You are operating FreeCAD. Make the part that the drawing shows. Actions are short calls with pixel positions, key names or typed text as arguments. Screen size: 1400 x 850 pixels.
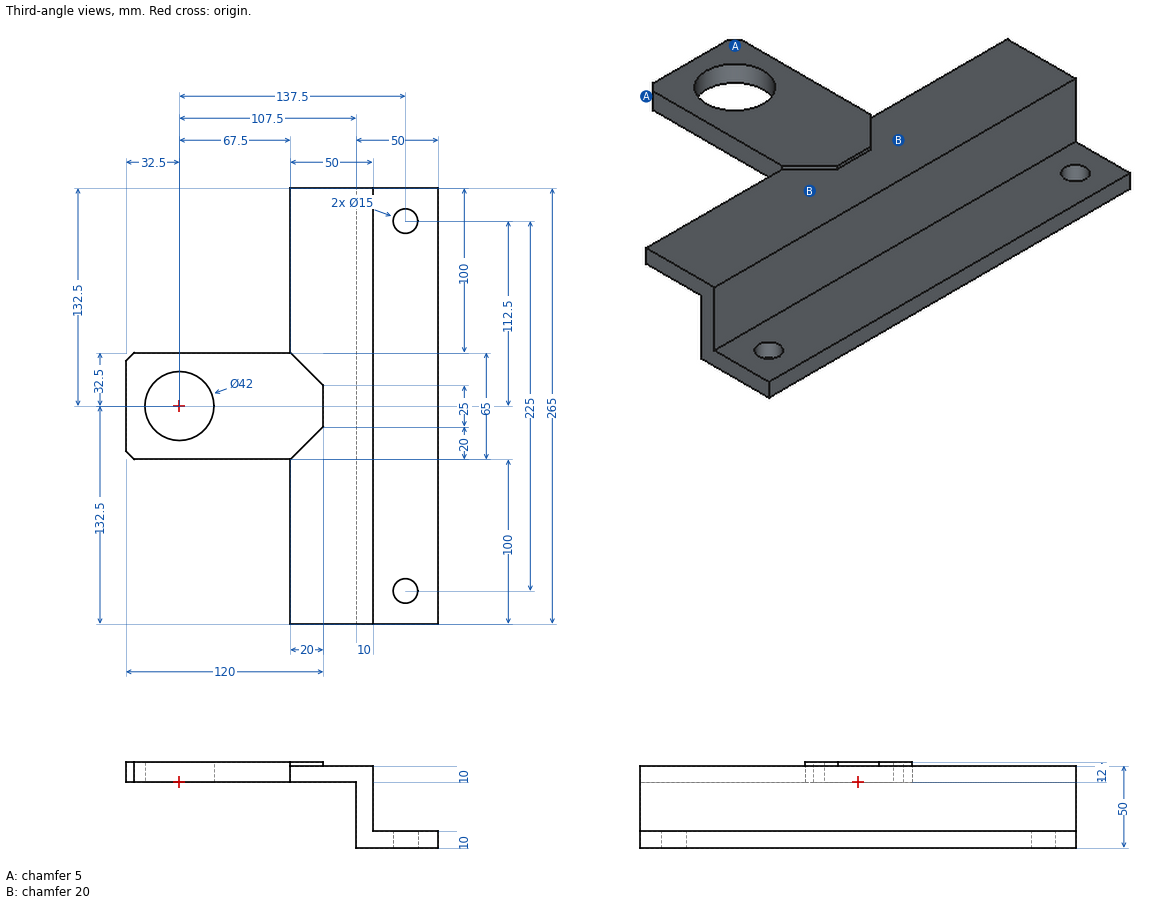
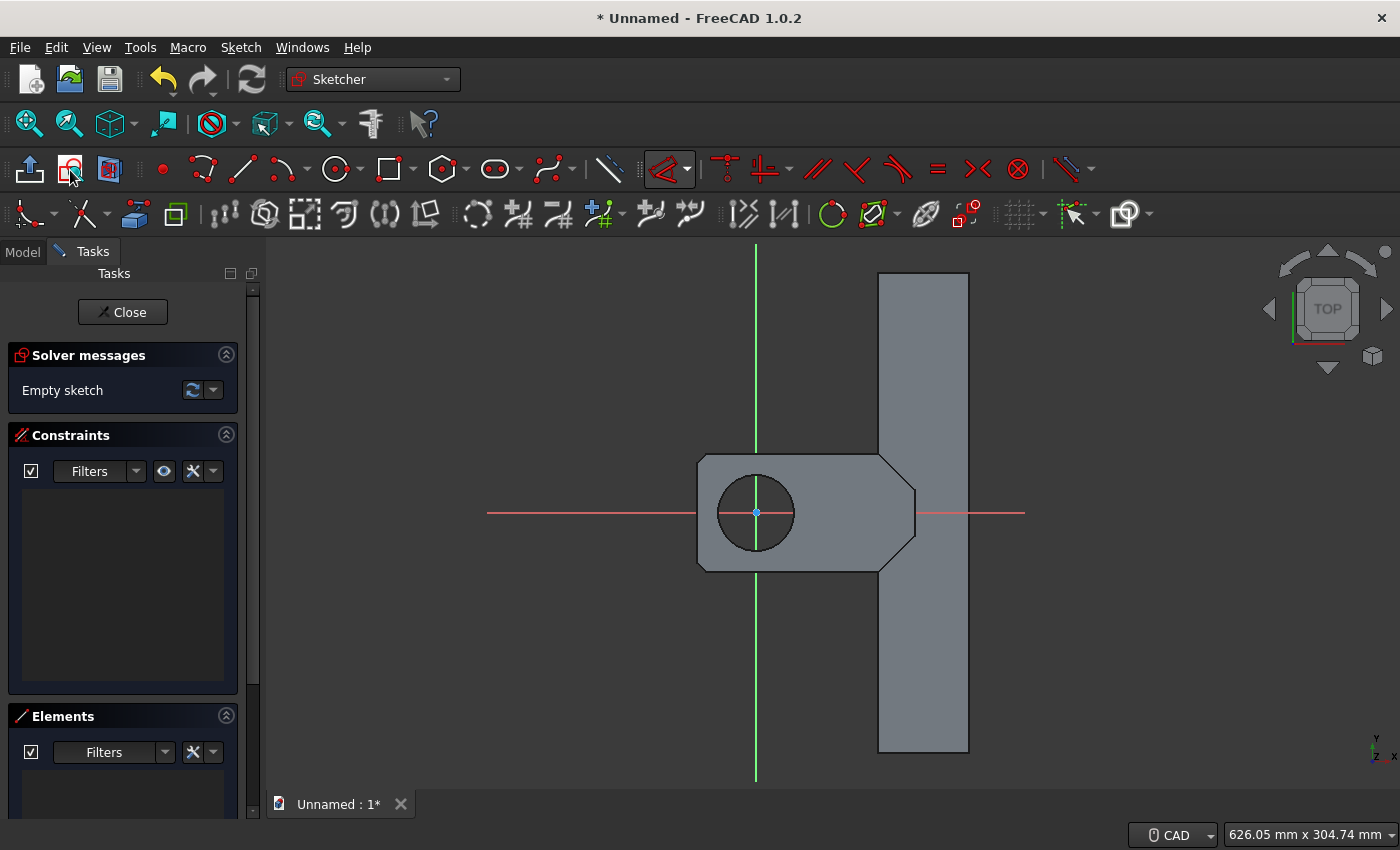
key(q)
key(s)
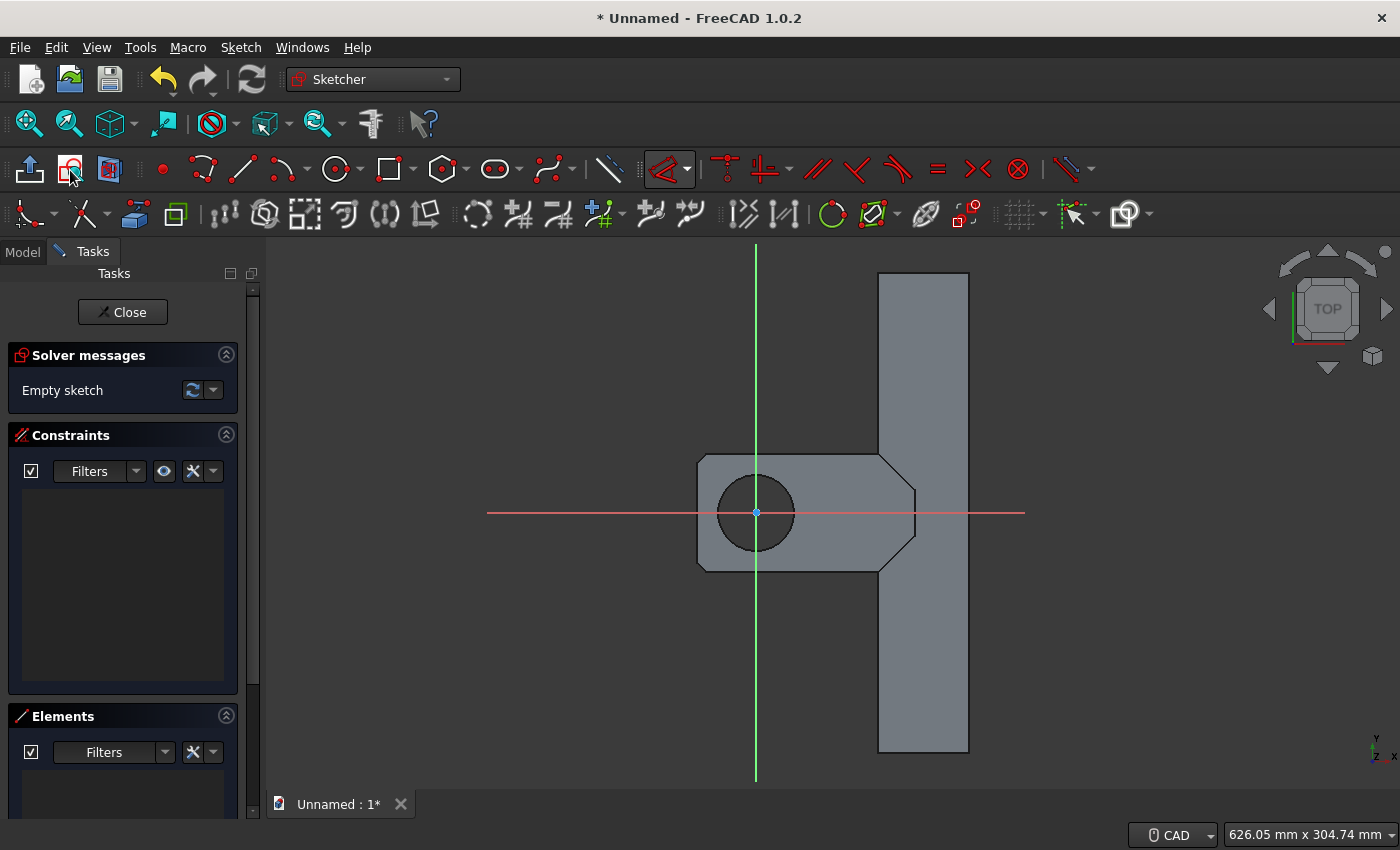
scroll(565, 513, down, 2)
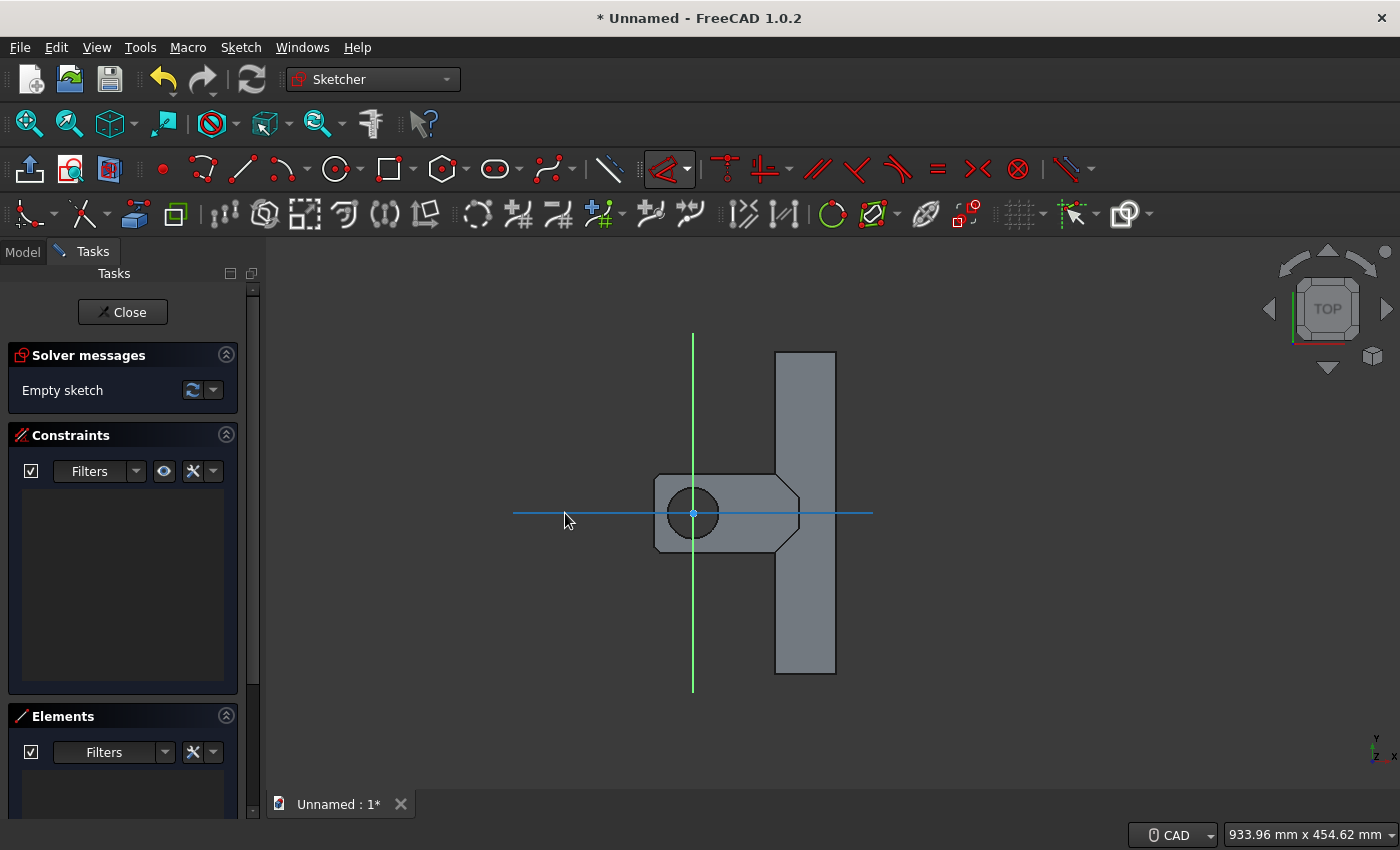
key(g)
key(r)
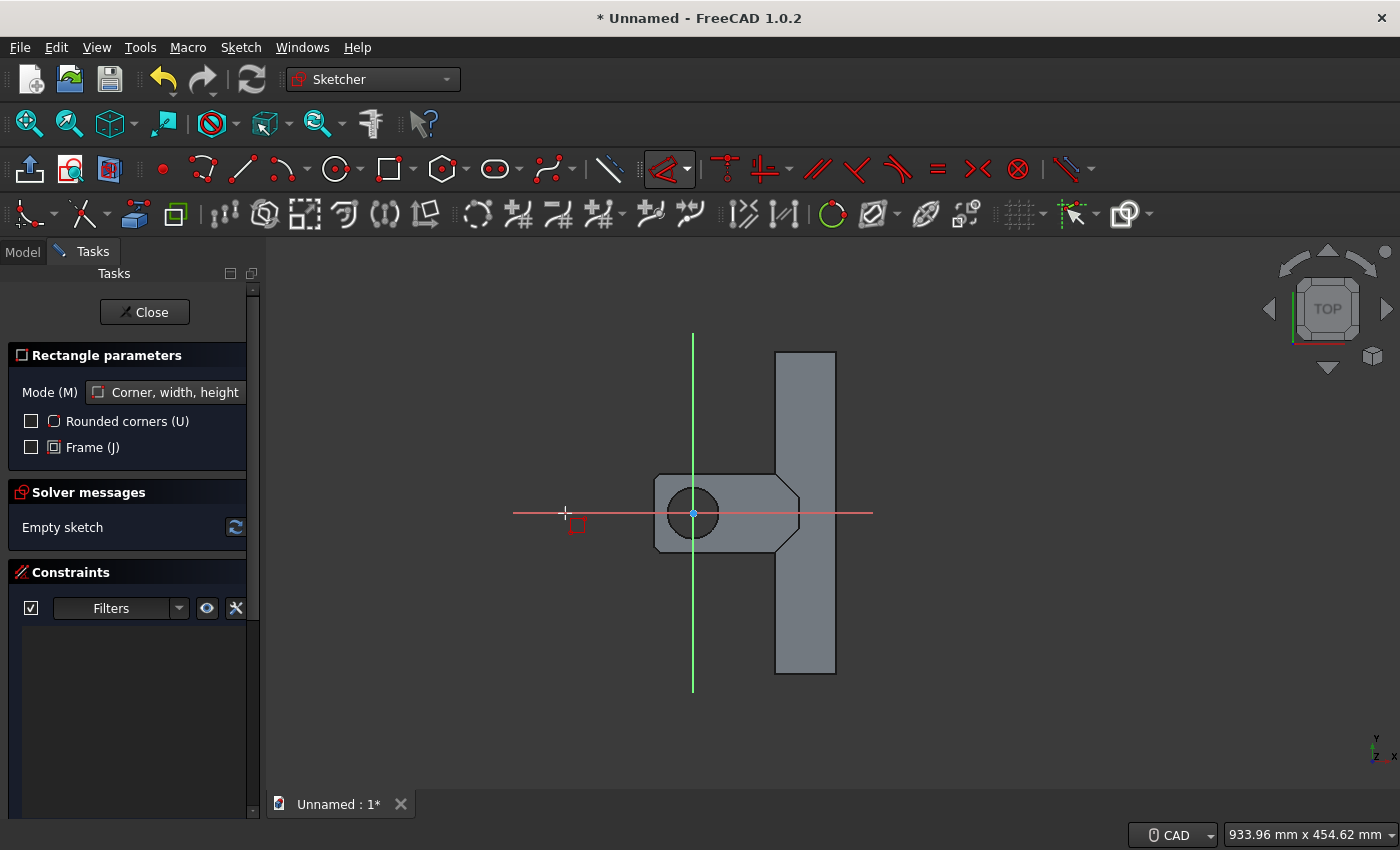
scroll(824, 352, up, 2)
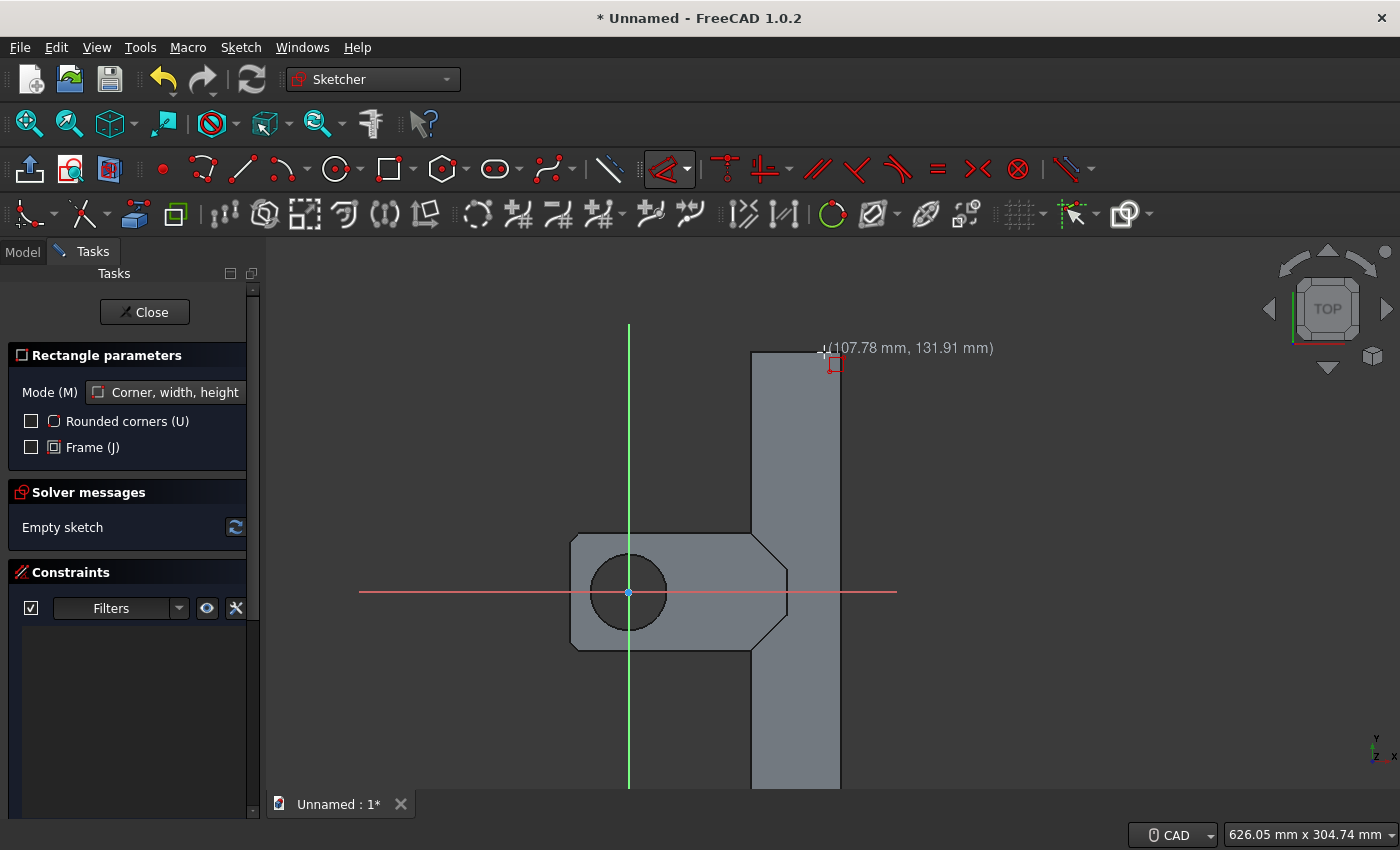
click(823, 352)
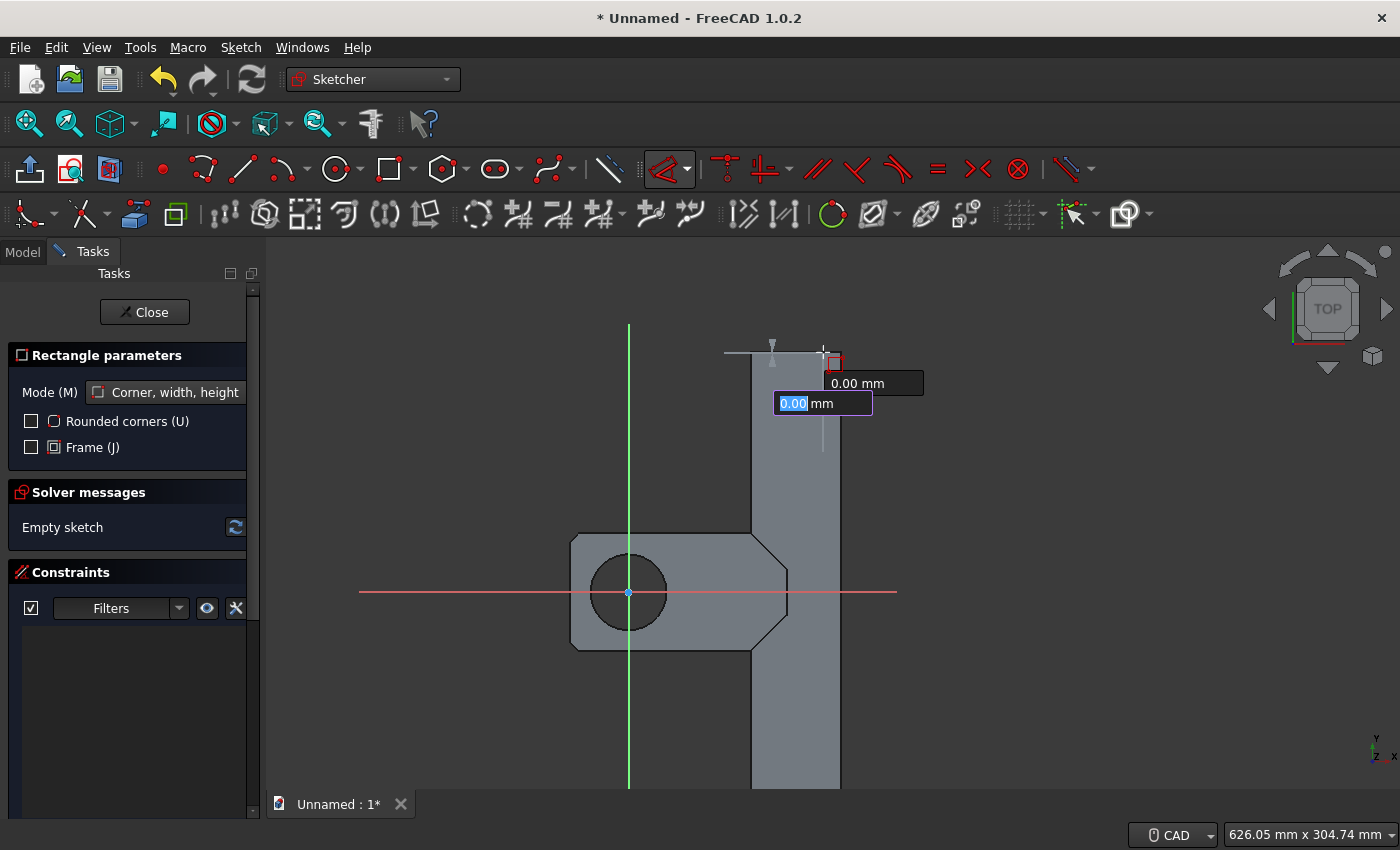
scroll(825, 352, down, 2)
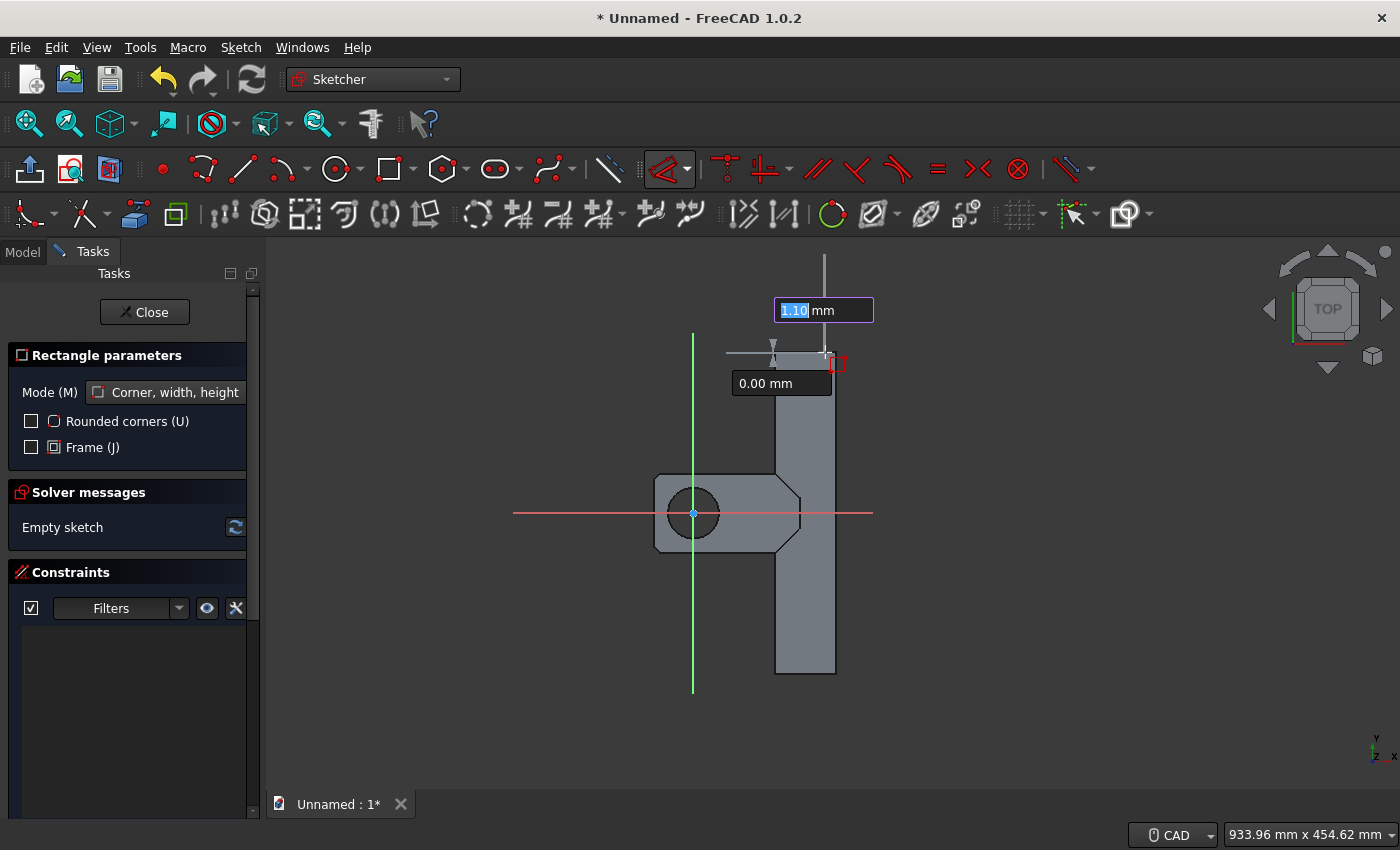
click(836, 674)
key(Escape)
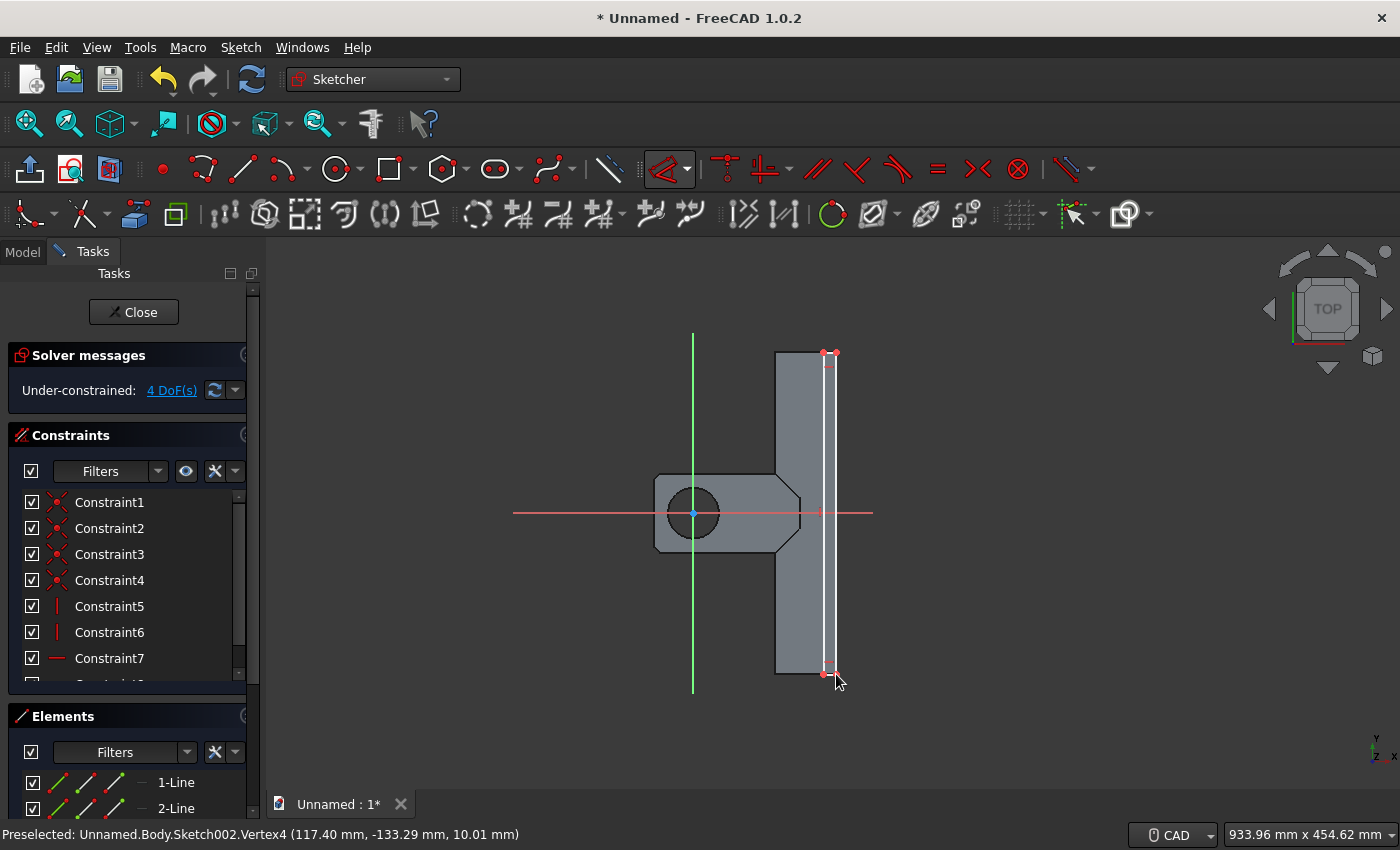
scroll(830, 675, up, 6)